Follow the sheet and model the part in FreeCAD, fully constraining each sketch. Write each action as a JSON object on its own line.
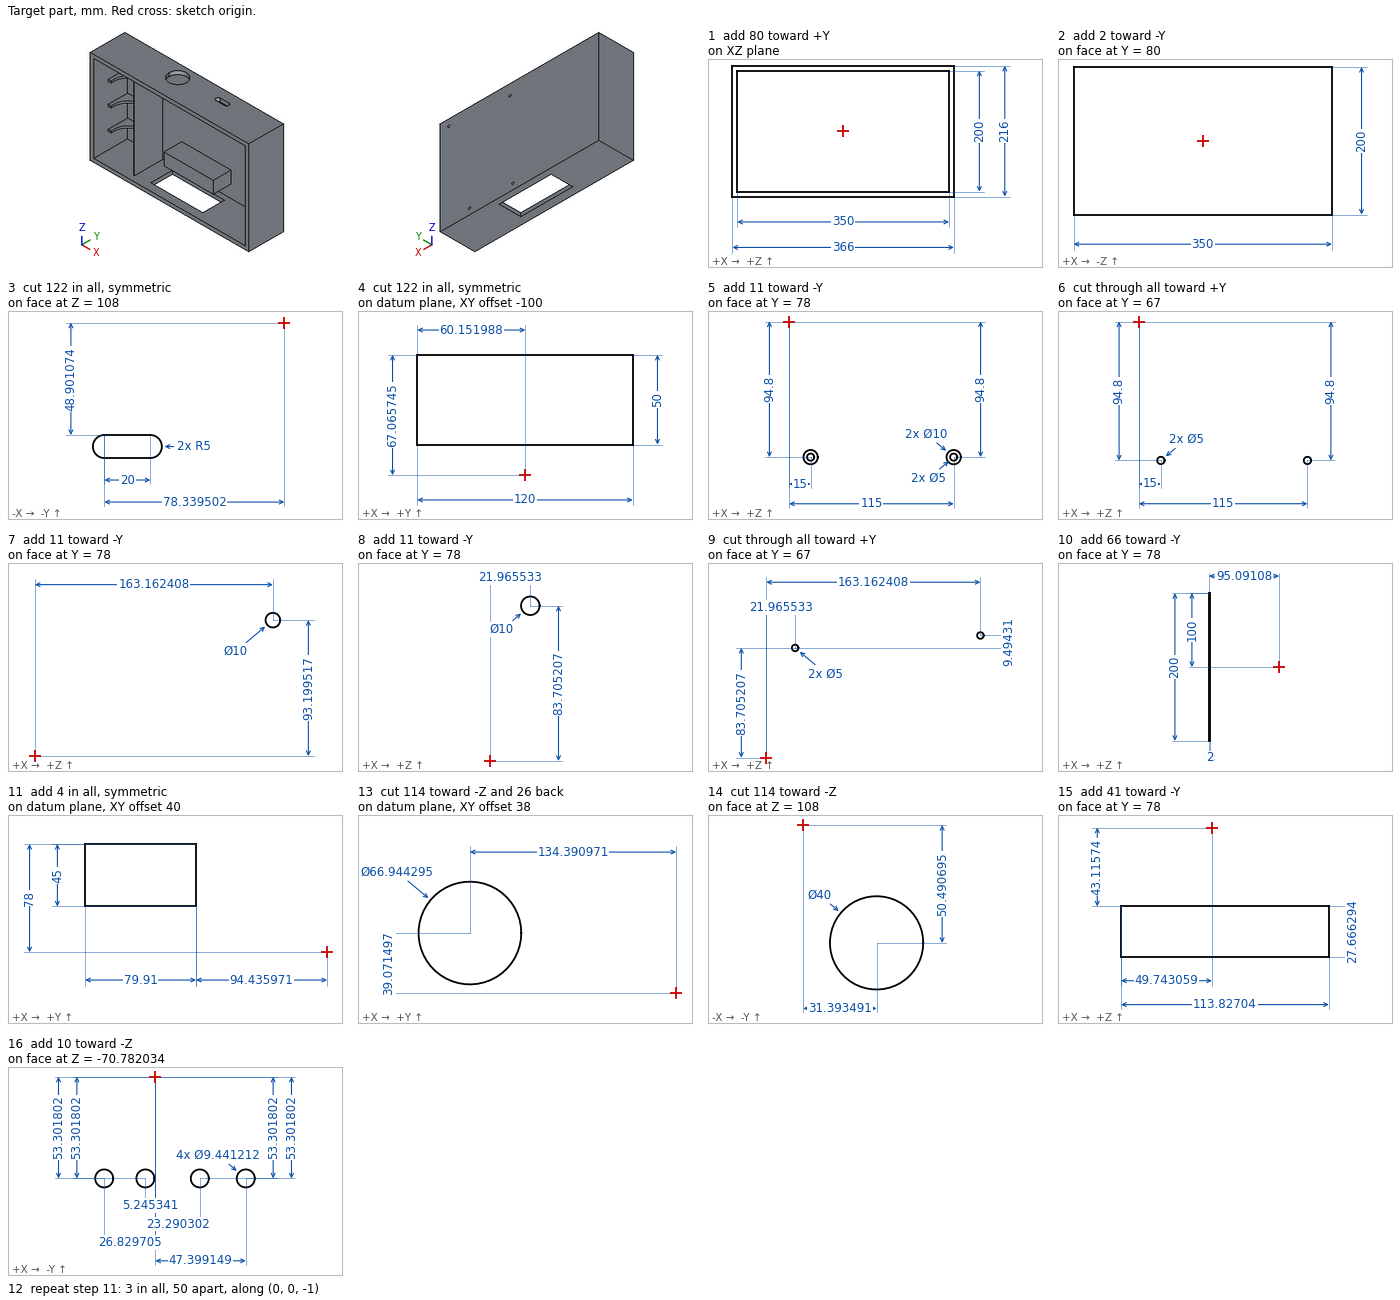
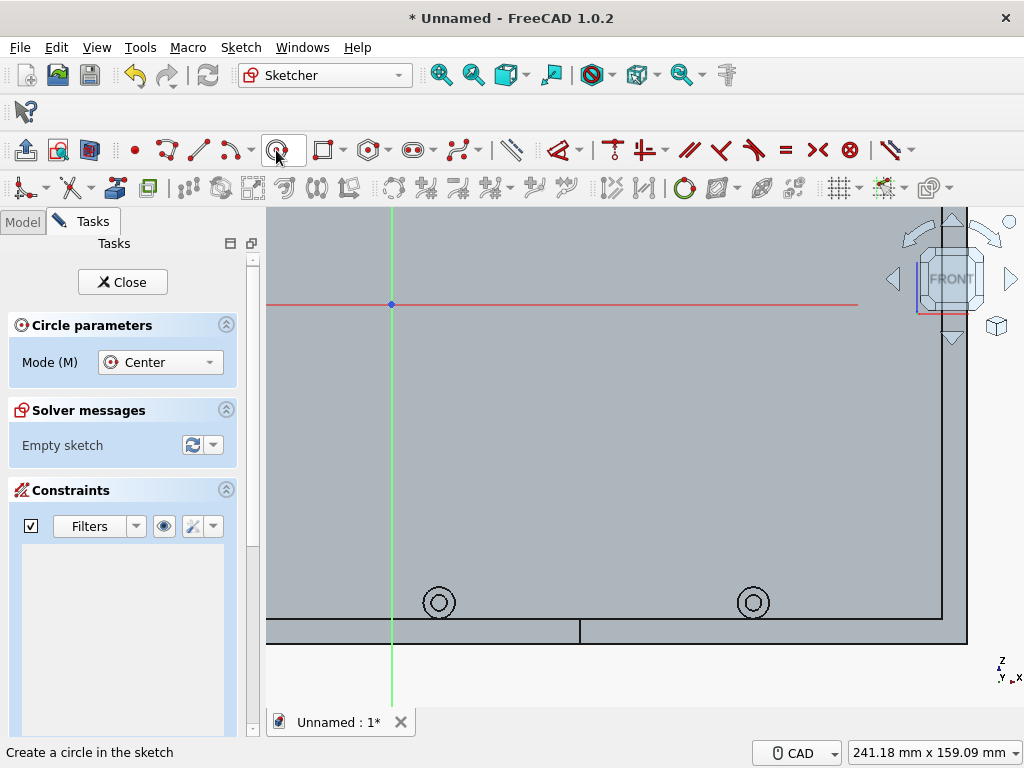
{"action": "scroll", "coordinate": [439, 603], "scroll_direction": "up", "scroll_amount": 6}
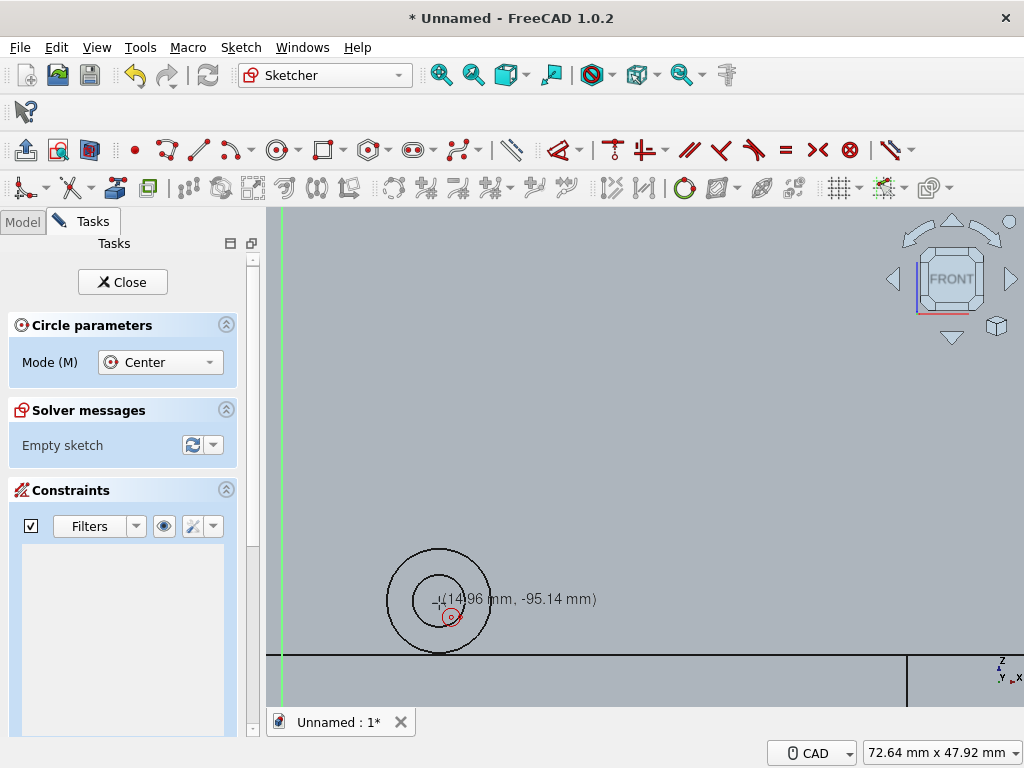
{"action": "left_click", "coordinate": [439, 601]}
{"action": "mouse_move", "coordinate": [457, 582]}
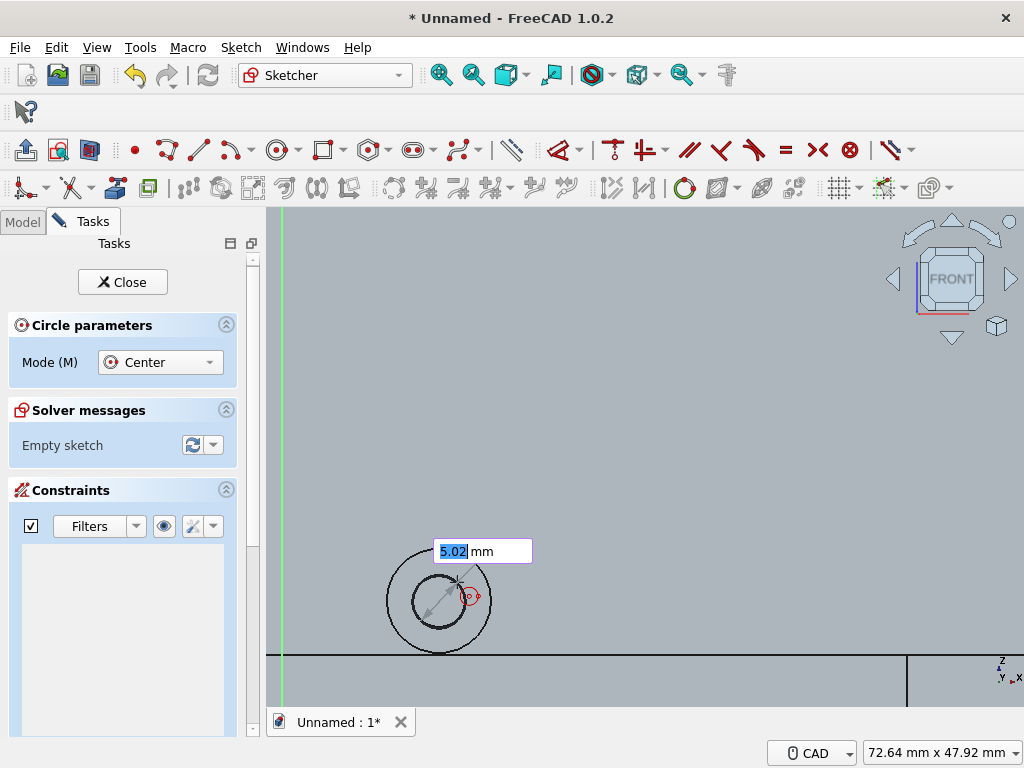
{"action": "type", "text": "5"}
{"action": "key", "text": "Return"}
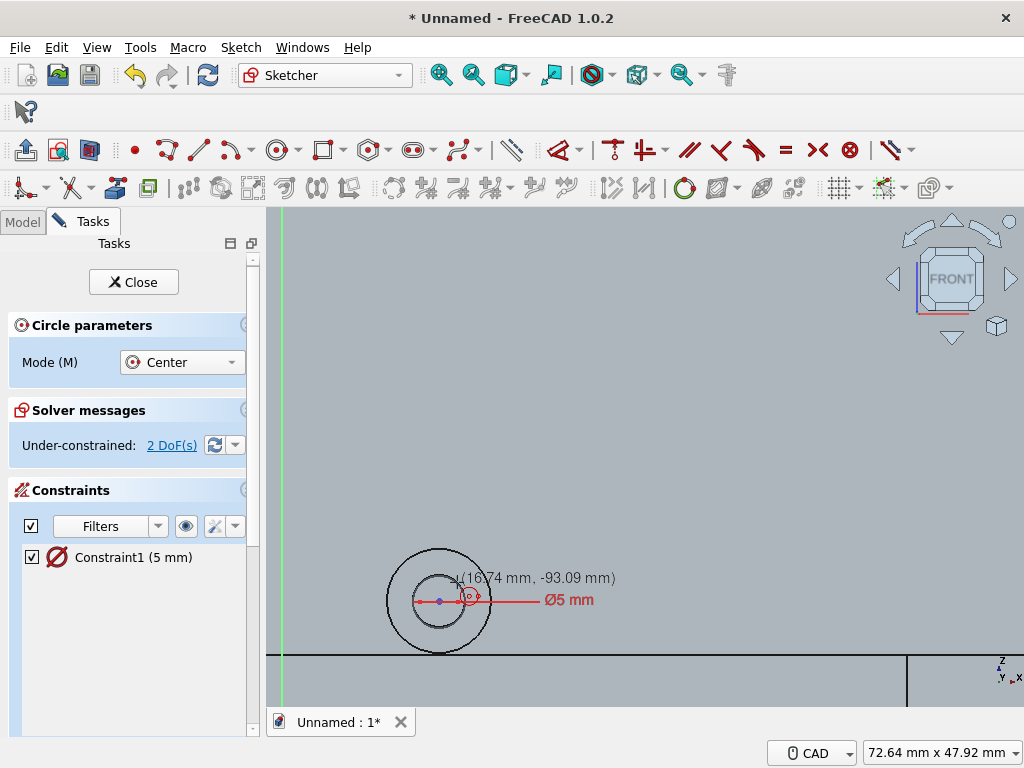
{"action": "scroll", "coordinate": [439, 603], "scroll_direction": "down", "scroll_amount": 6}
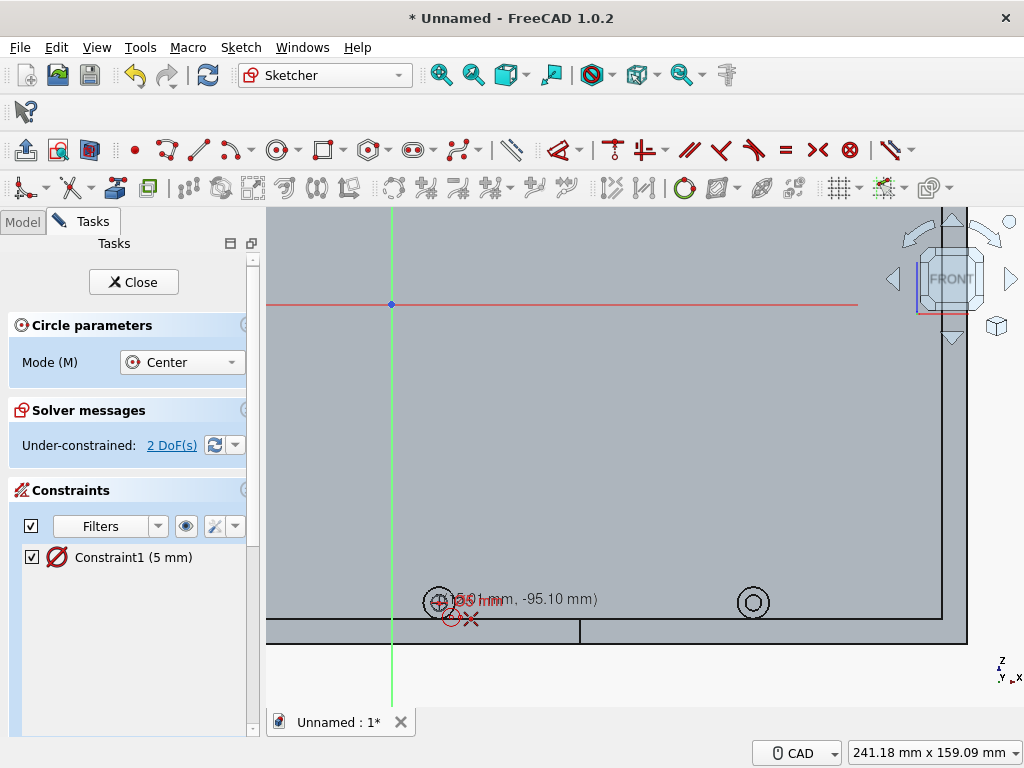
{"action": "scroll", "coordinate": [753, 603], "scroll_direction": "up", "scroll_amount": 6}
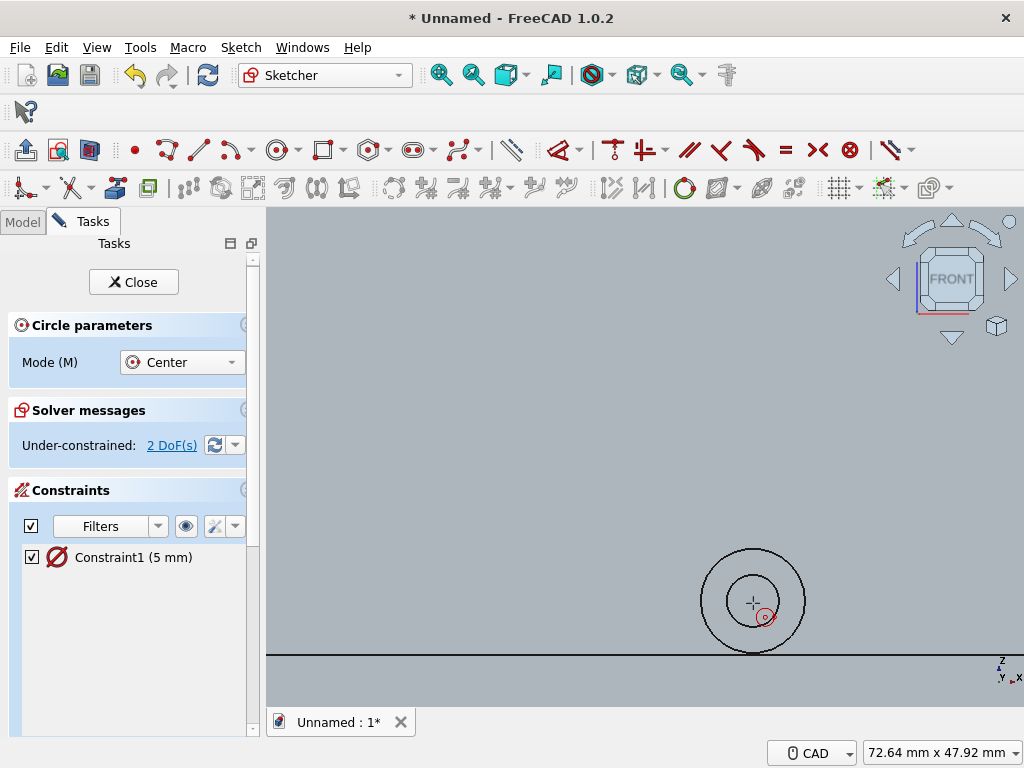
{"action": "left_click", "coordinate": [753, 601]}
{"action": "mouse_move", "coordinate": [771, 582]}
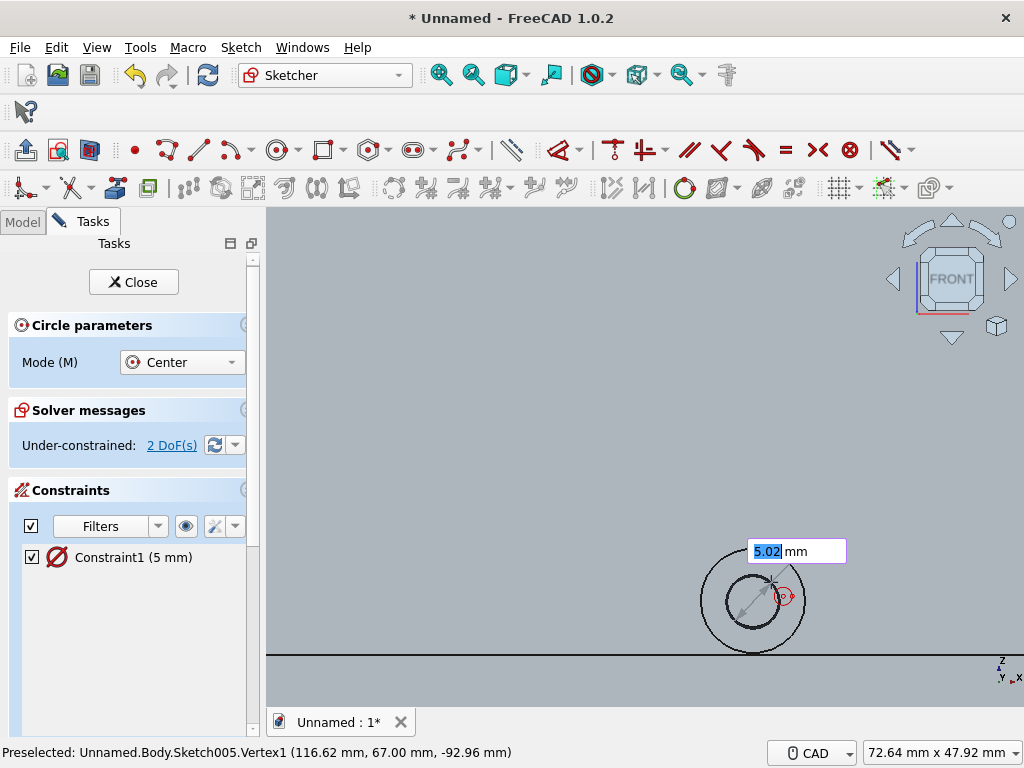
{"action": "type", "text": "5"}
{"action": "key", "text": "Return"}
{"action": "key", "text": "Escape"}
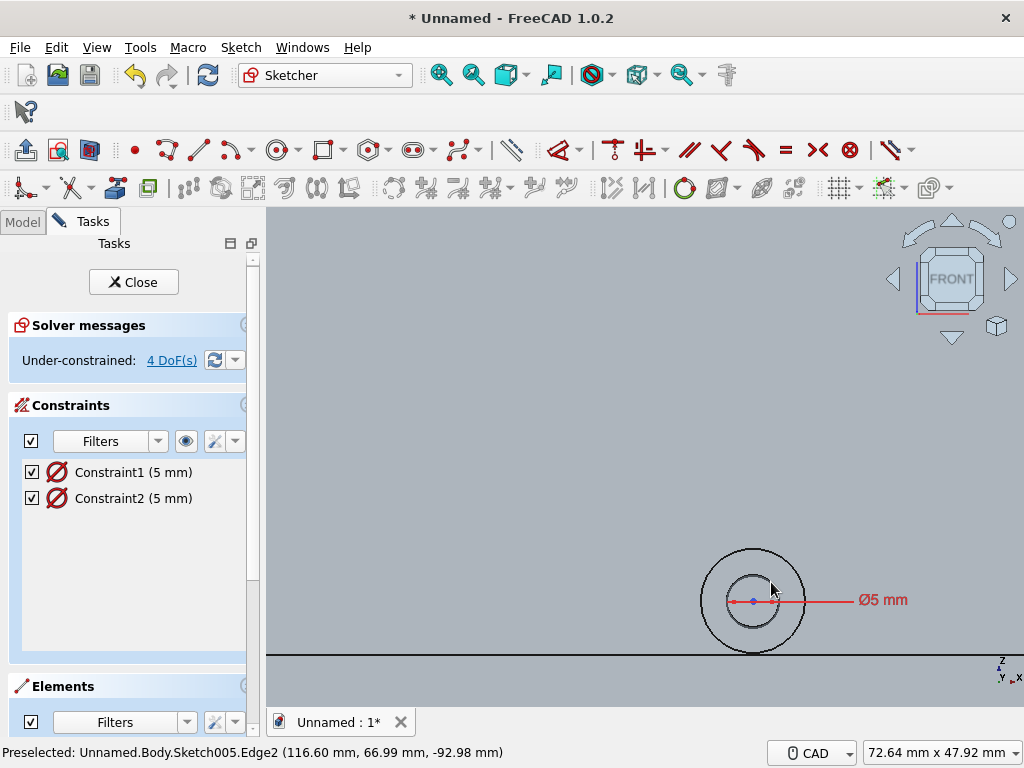
{"action": "left_click", "coordinate": [558, 150]}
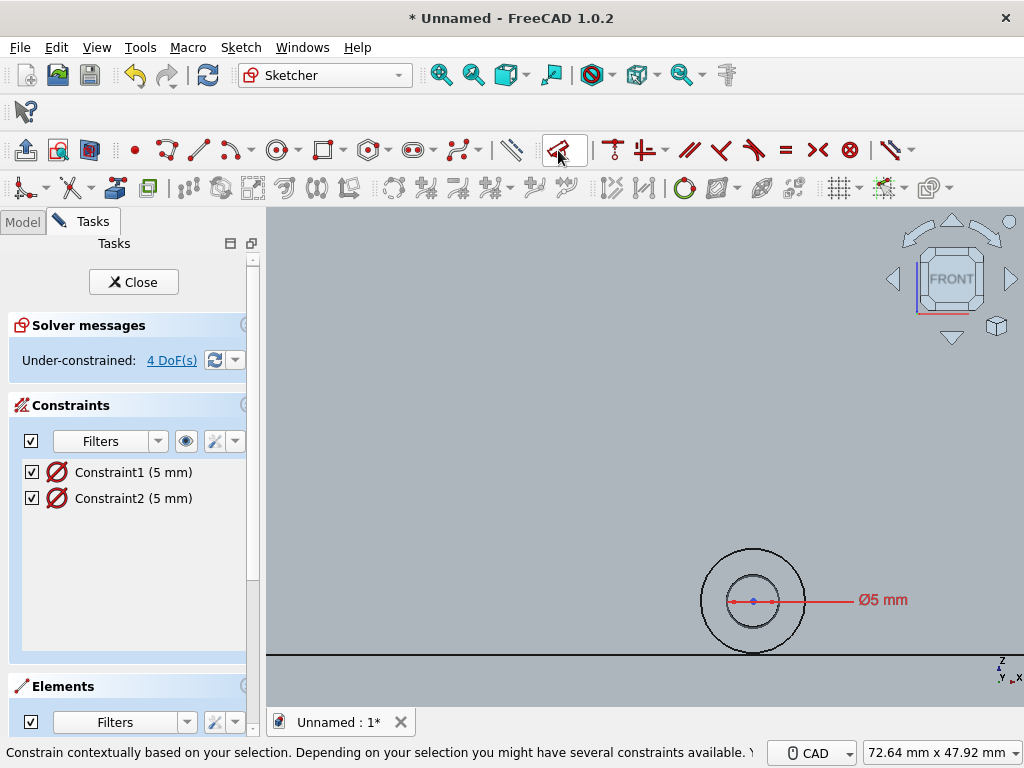
{"action": "scroll", "coordinate": [753, 603], "scroll_direction": "down", "scroll_amount": 6}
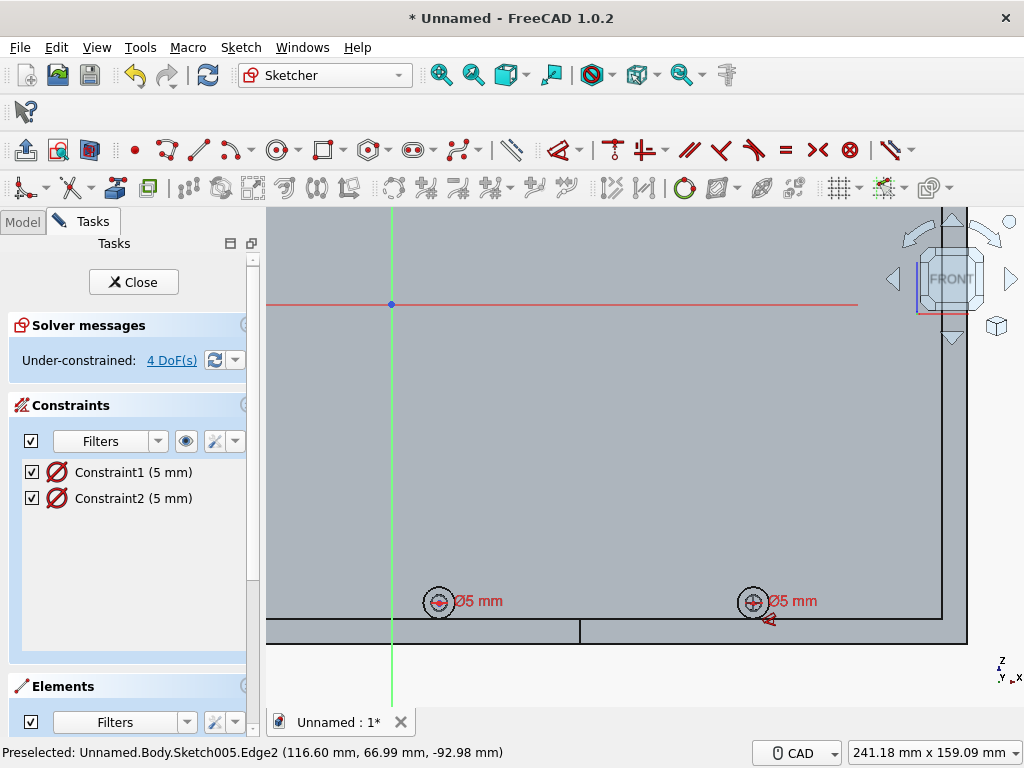
{"action": "left_click", "coordinate": [439, 603]}
{"action": "left_click", "coordinate": [416, 271]}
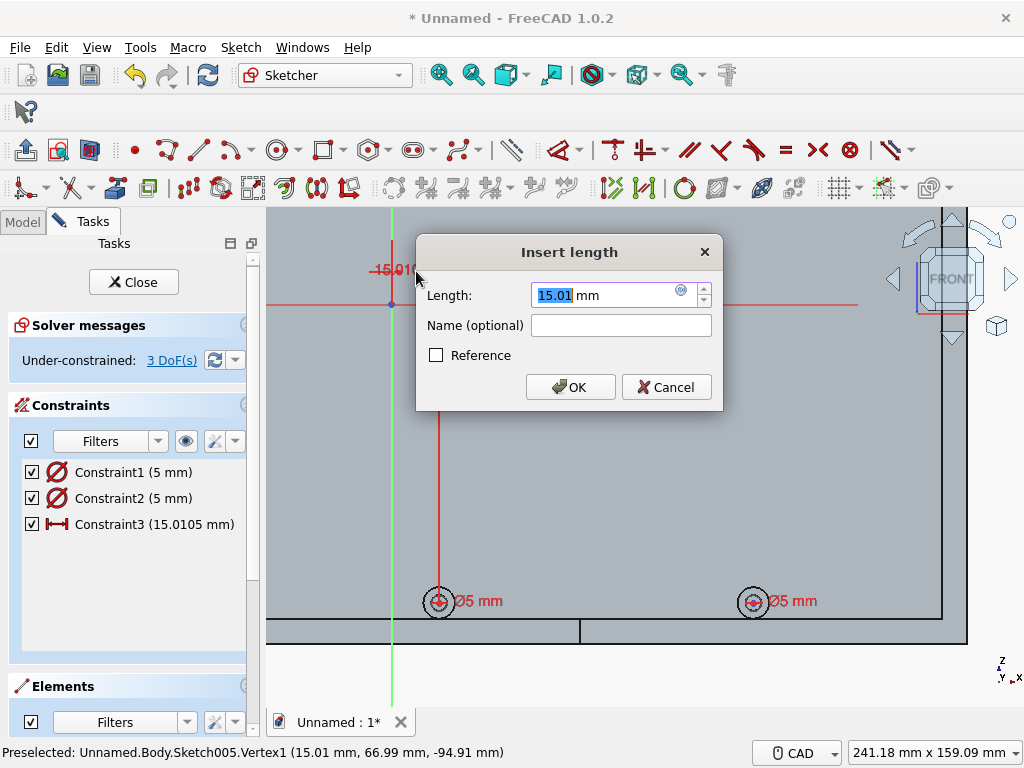
{"action": "type", "text": "15"}
{"action": "key", "text": "Return"}